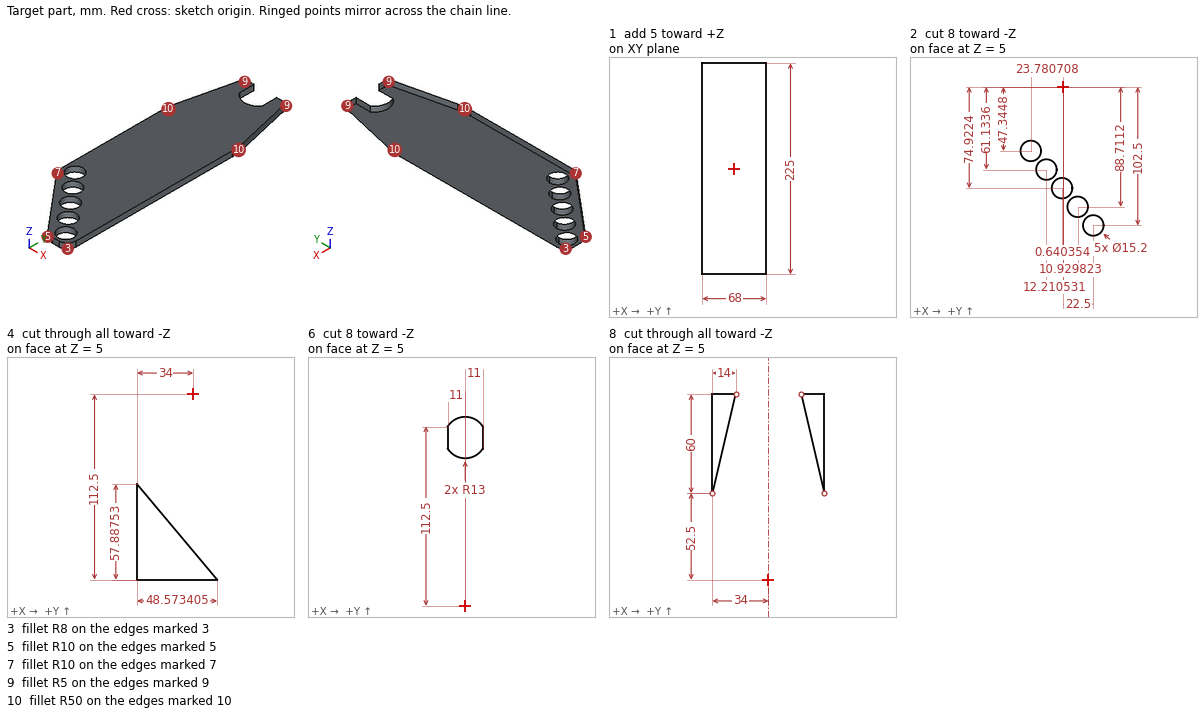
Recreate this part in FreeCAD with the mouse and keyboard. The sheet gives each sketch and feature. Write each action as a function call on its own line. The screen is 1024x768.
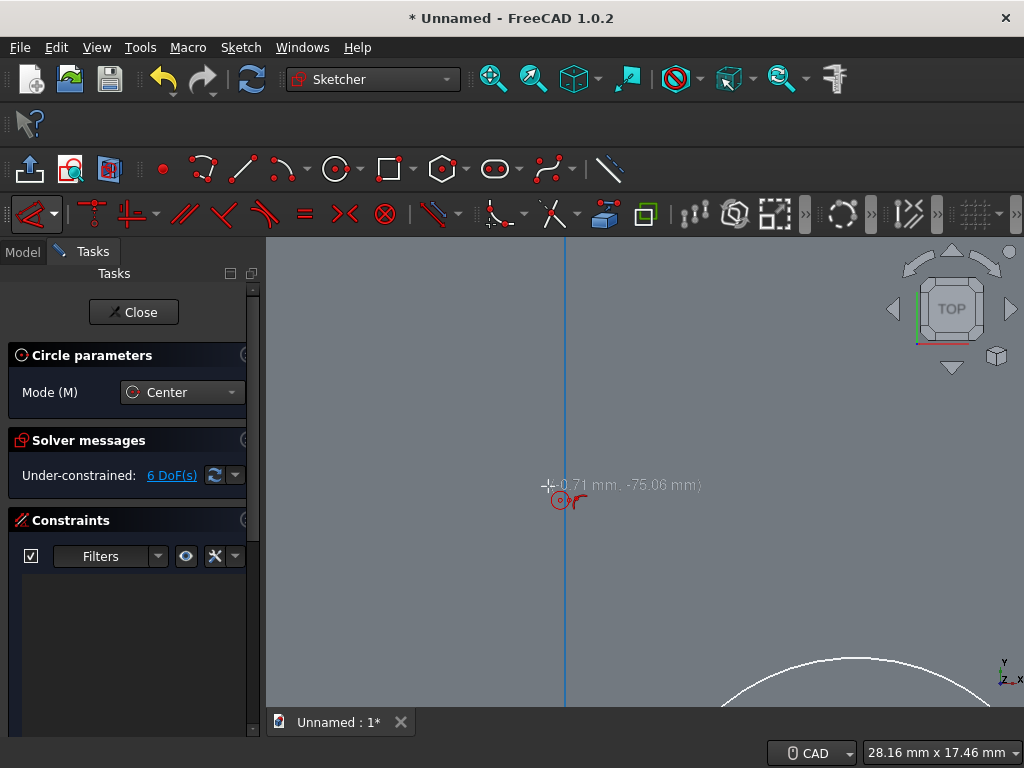
click(547, 486)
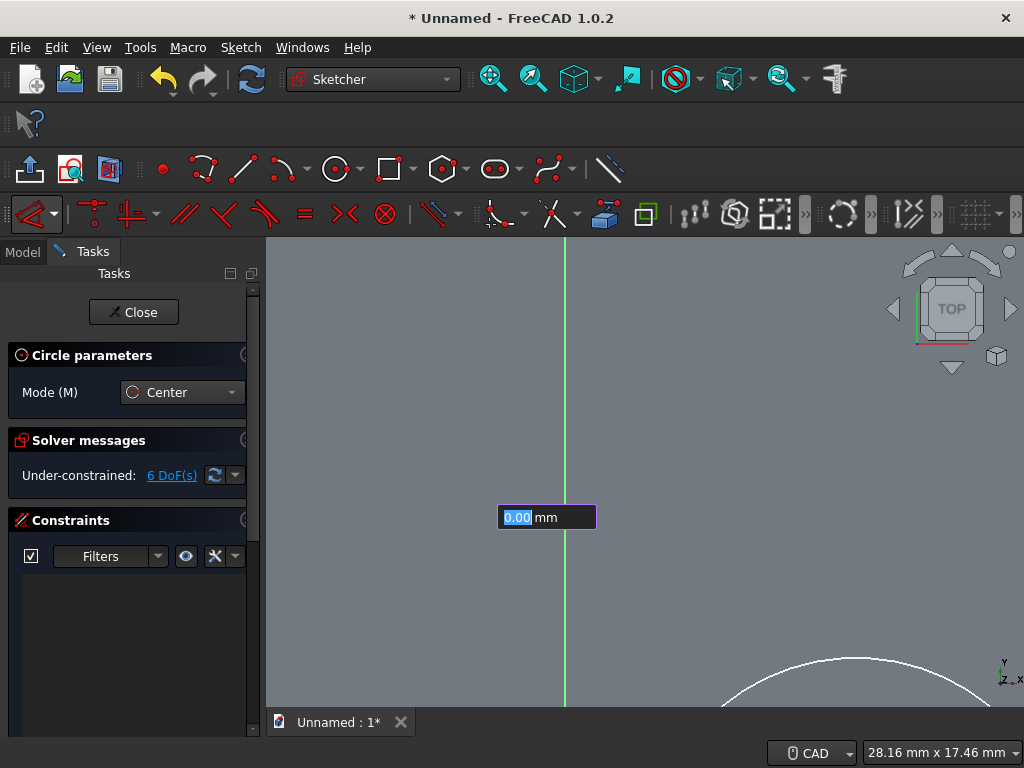
scroll(579, 524, down, 12)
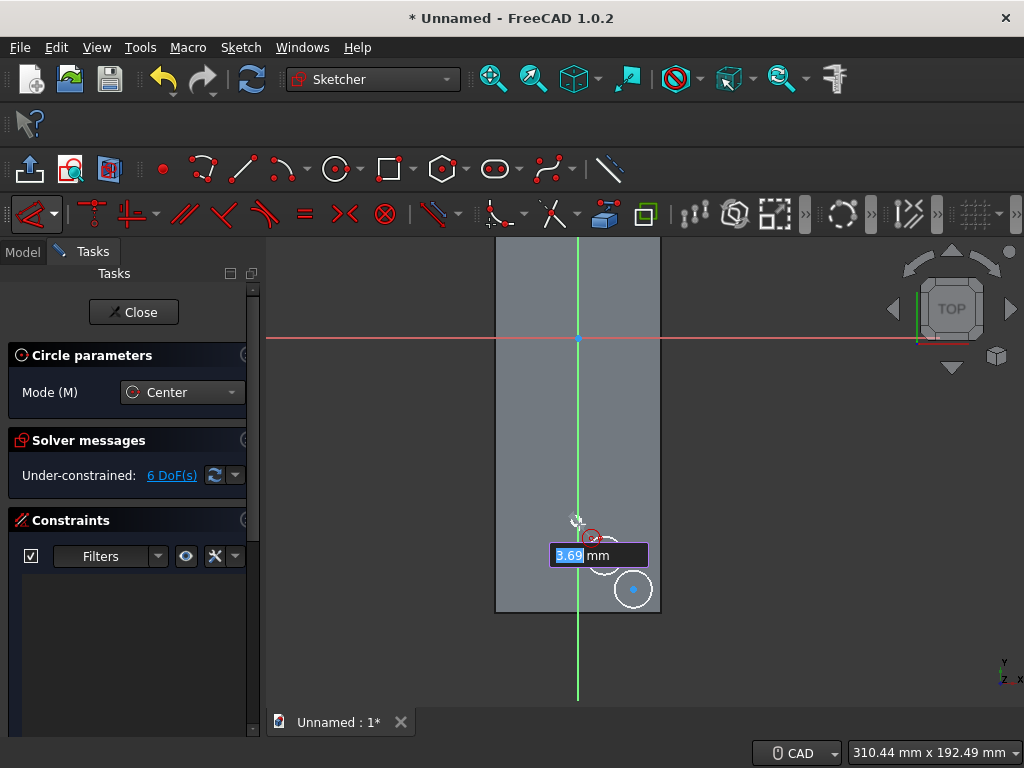
scroll(590, 508, up, 2)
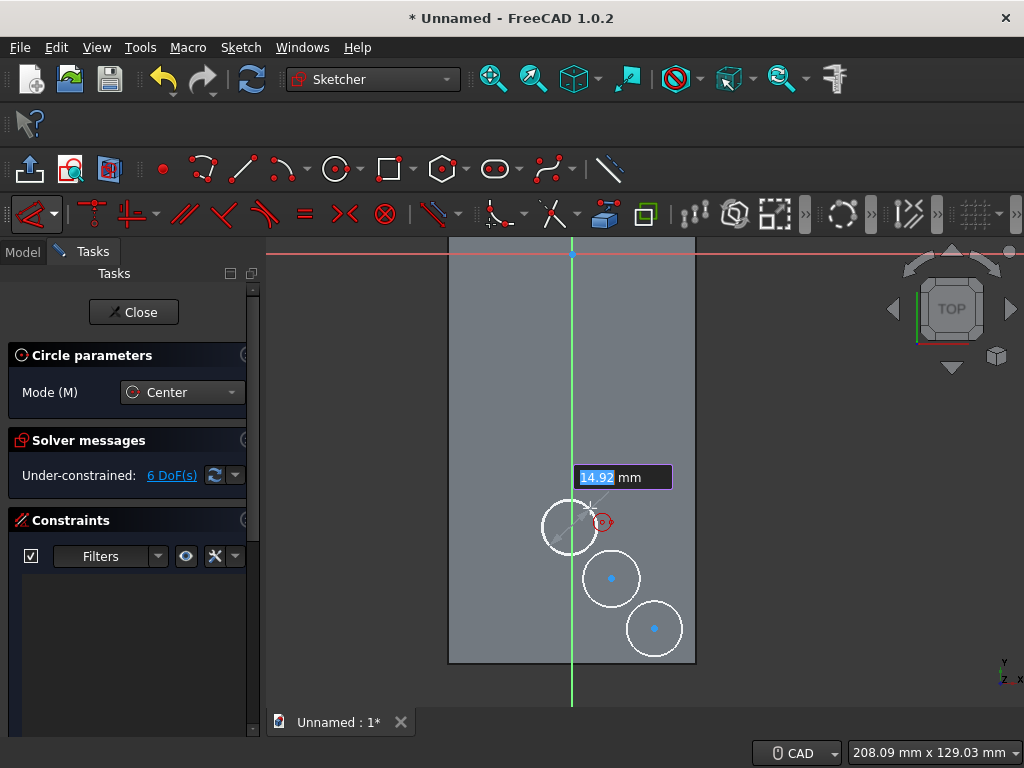
click(589, 508)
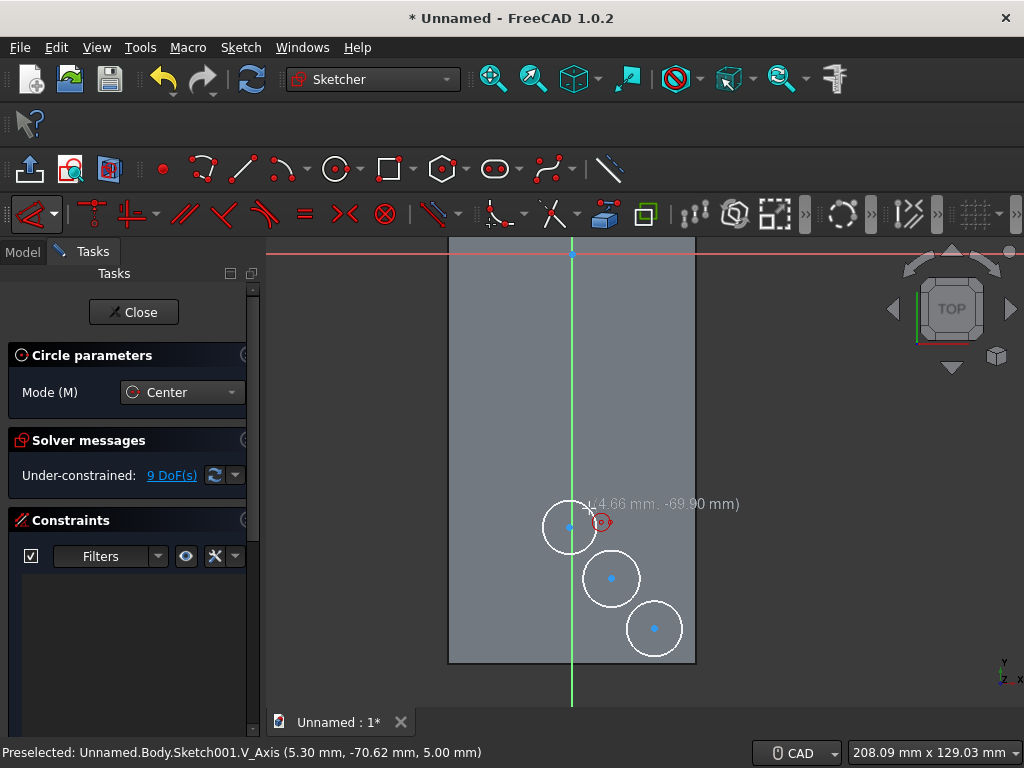
click(528, 477)
click(547, 458)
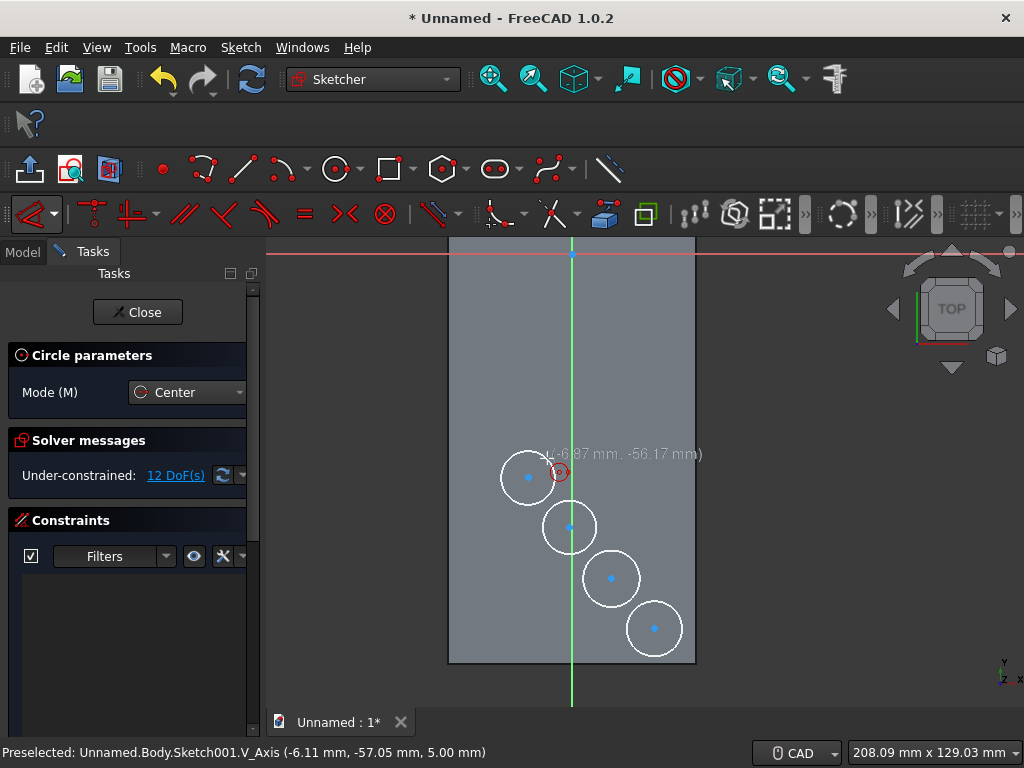
click(485, 427)
click(505, 407)
key(Escape)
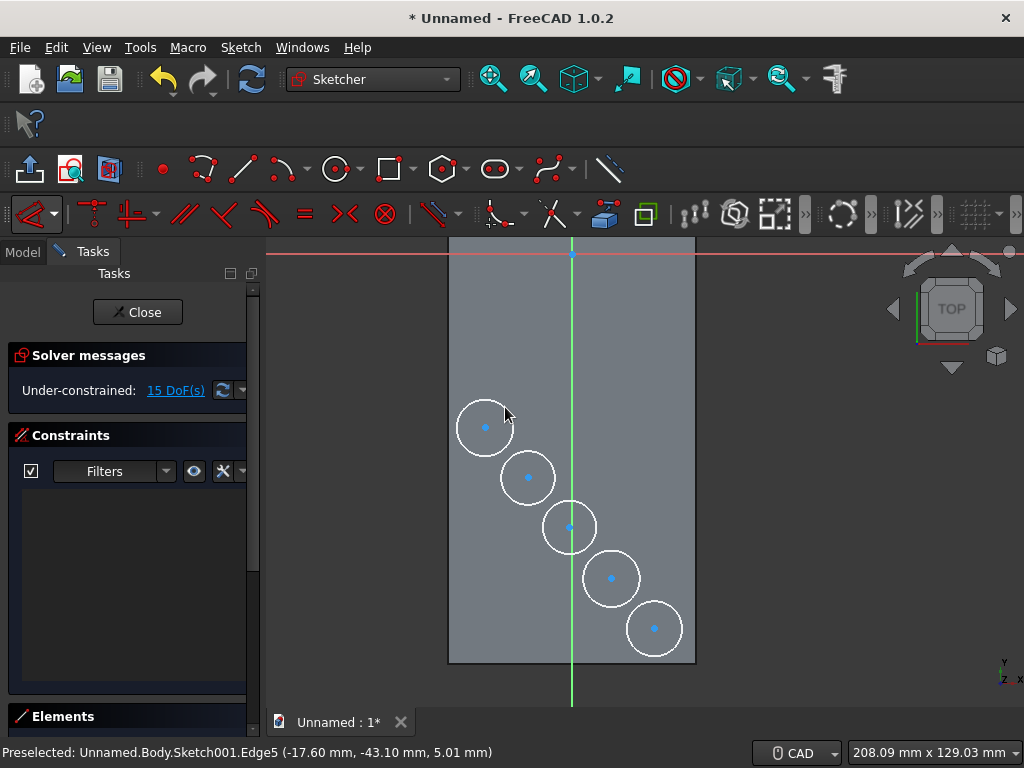
click(674, 609)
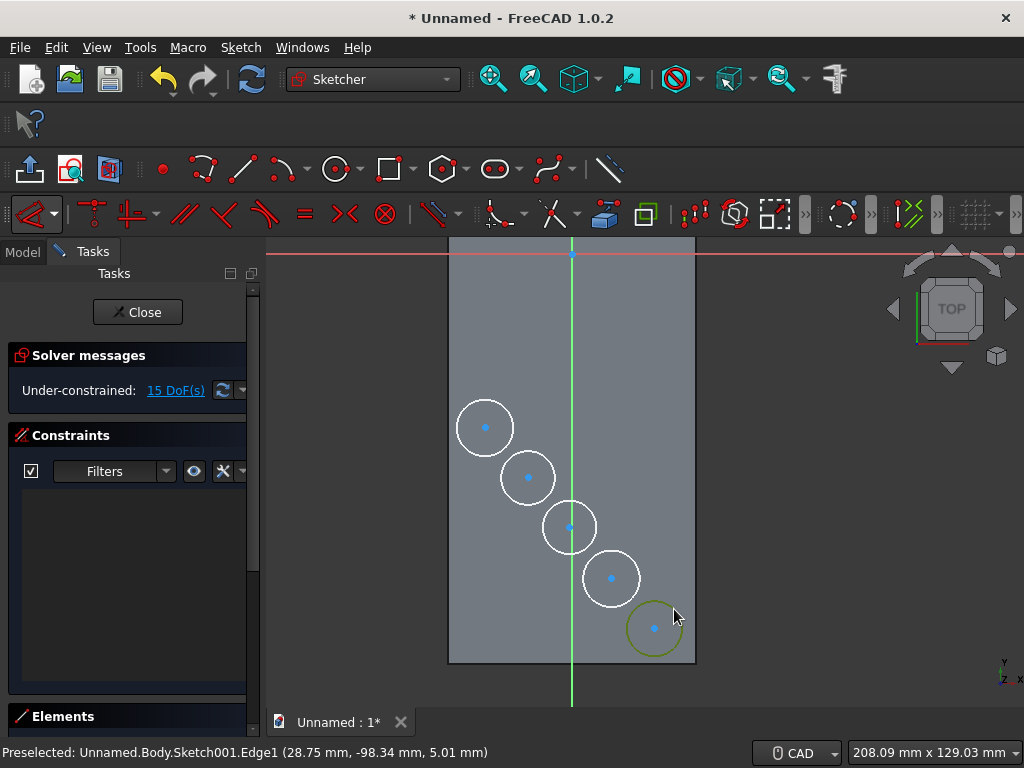
click(631, 559)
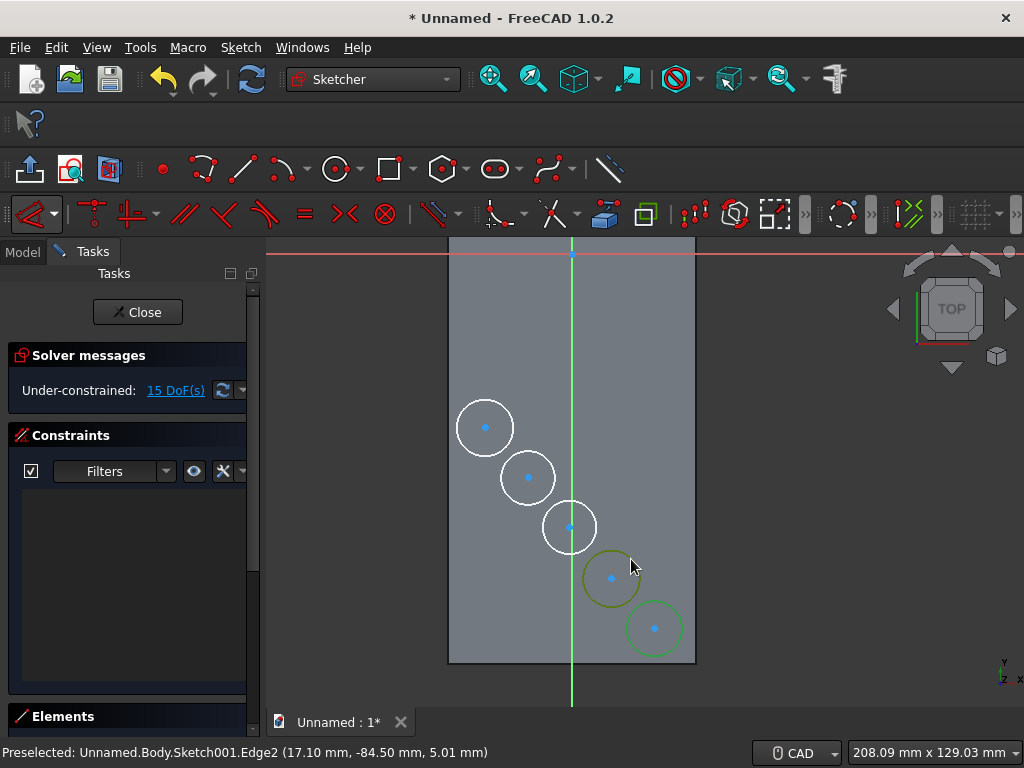
click(588, 508)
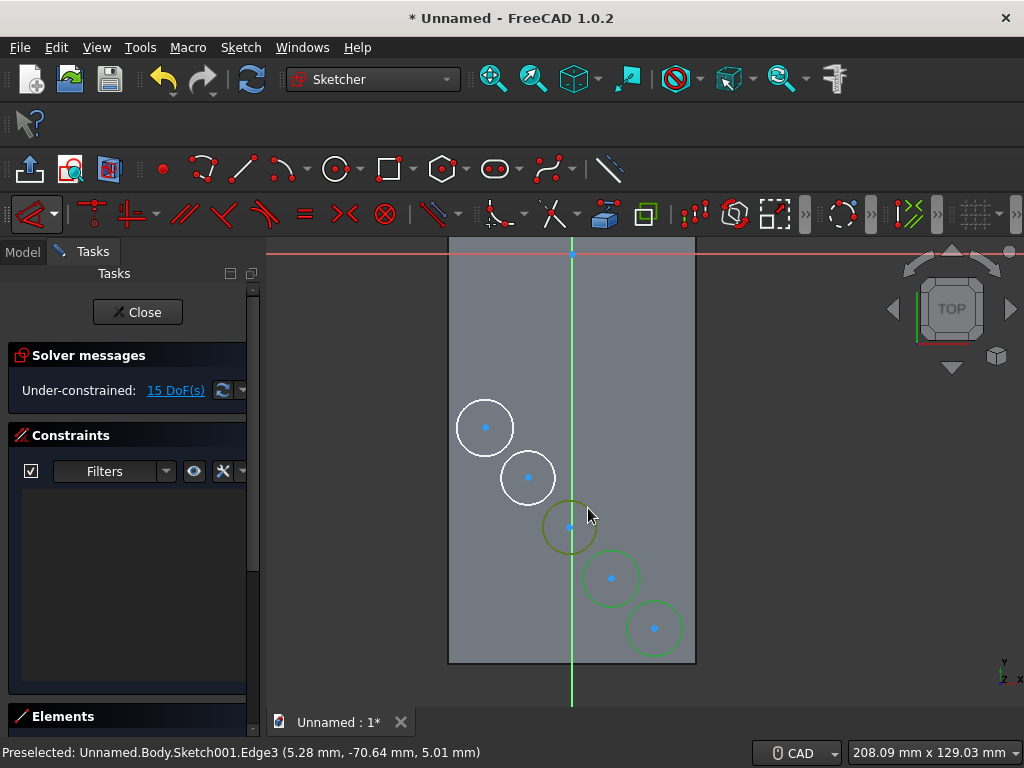
click(547, 459)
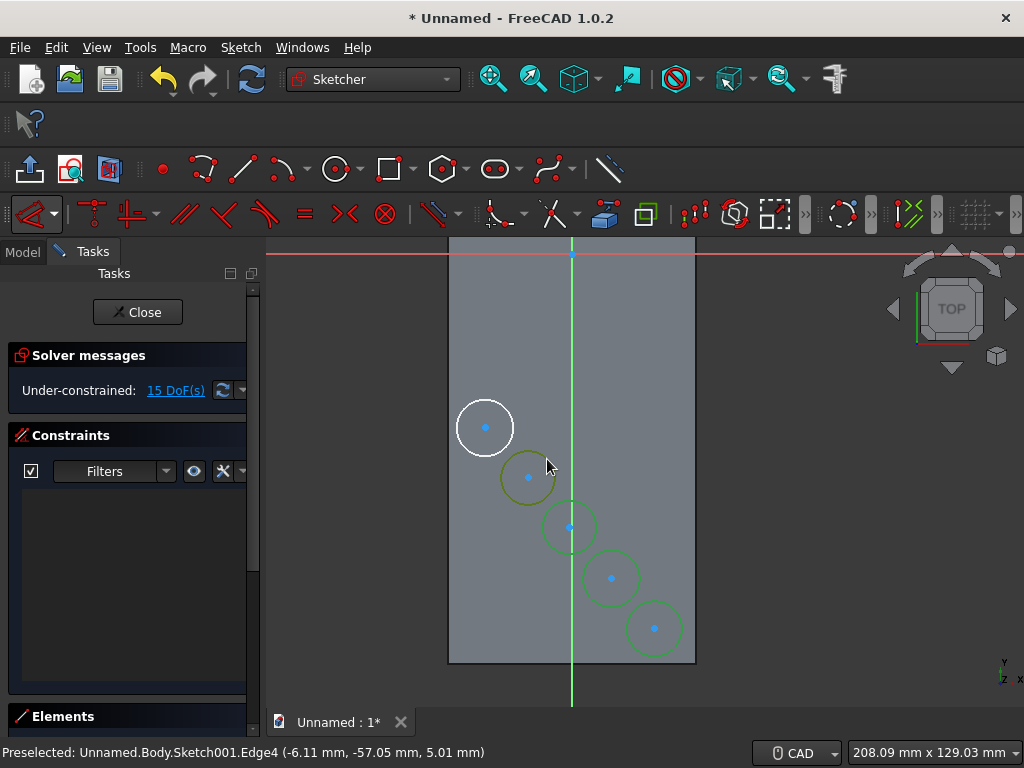
click(505, 408)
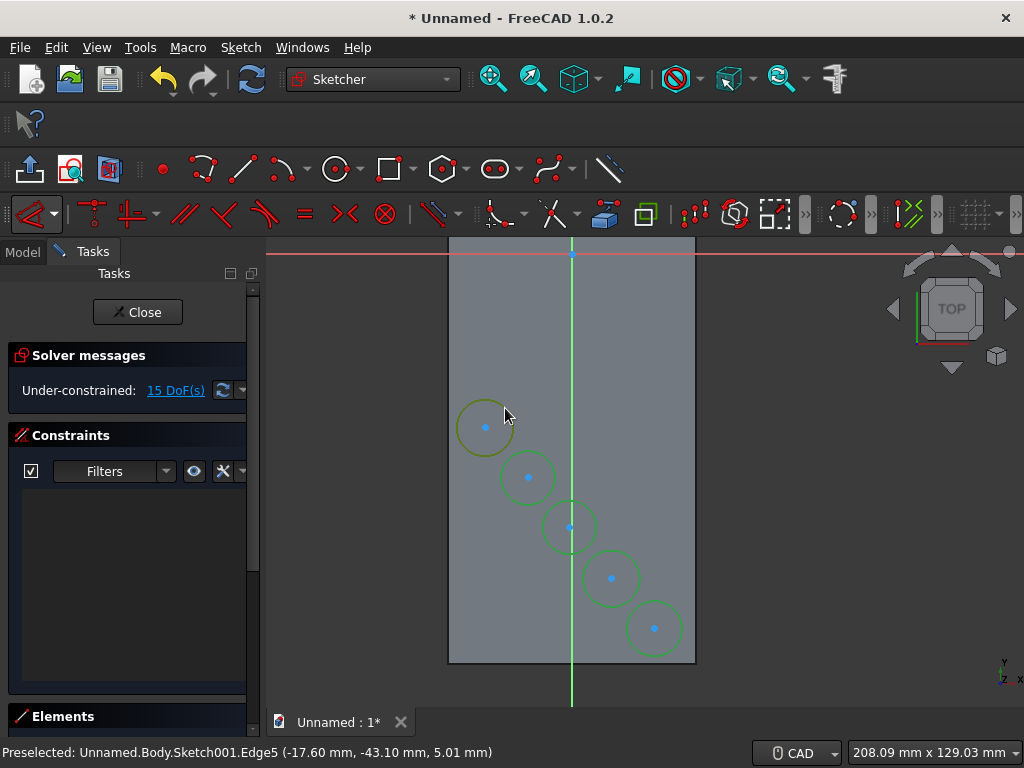
key(e)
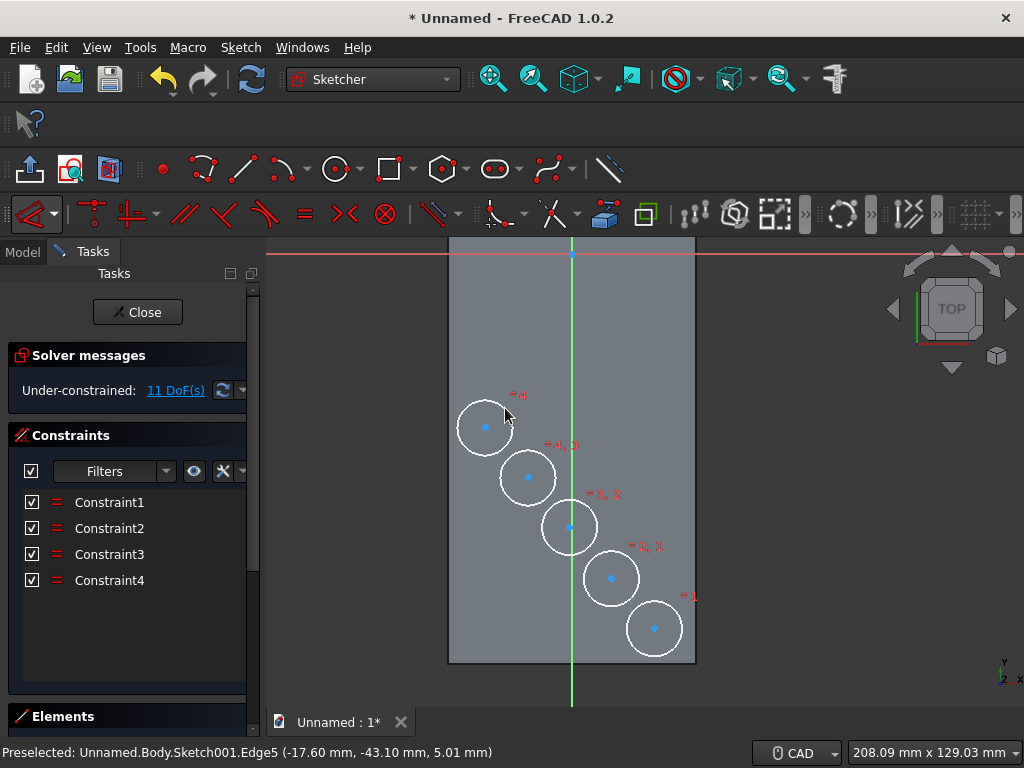
click(30, 214)